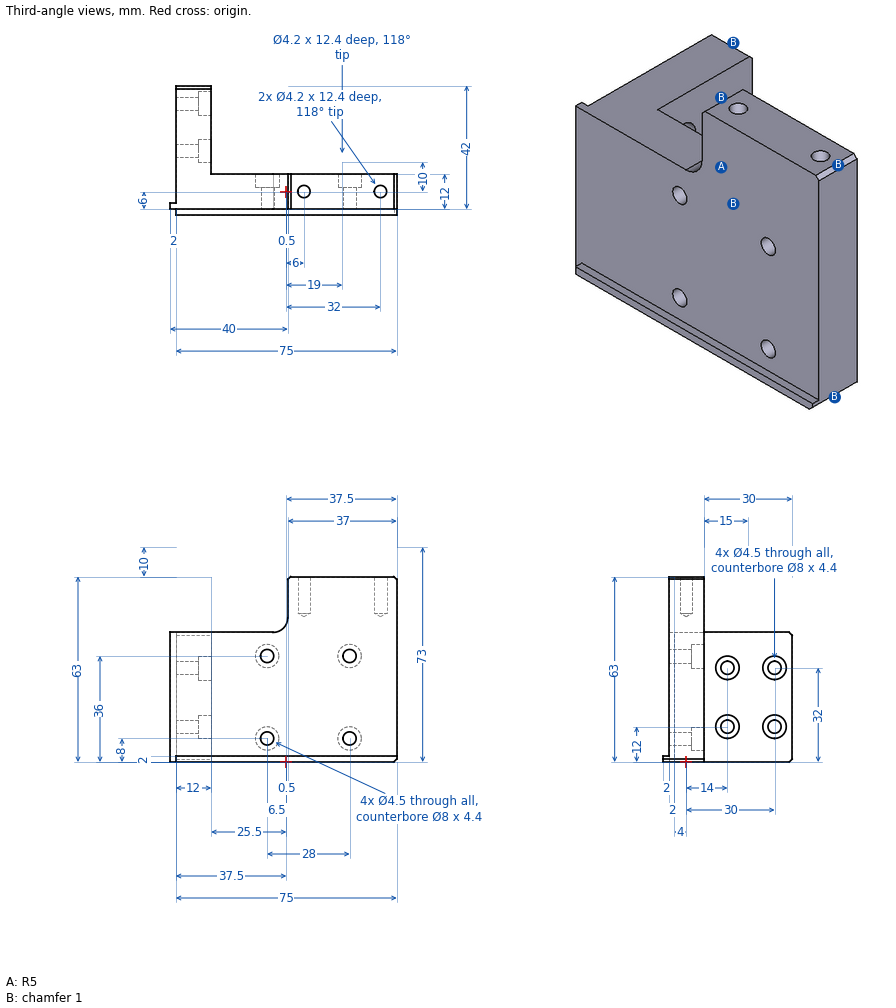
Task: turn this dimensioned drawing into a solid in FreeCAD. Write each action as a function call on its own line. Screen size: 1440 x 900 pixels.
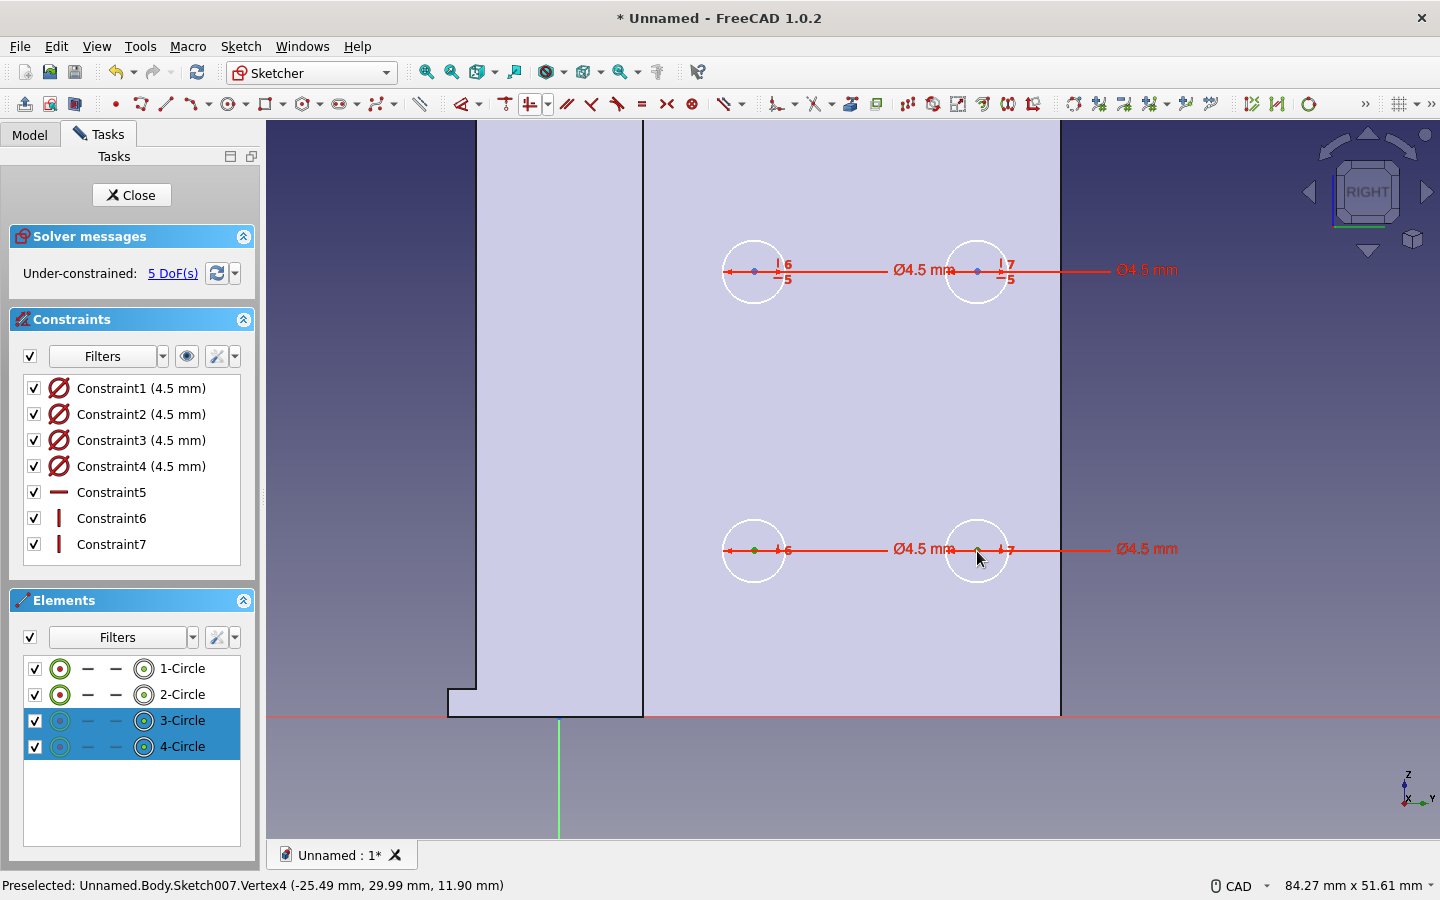
key(h)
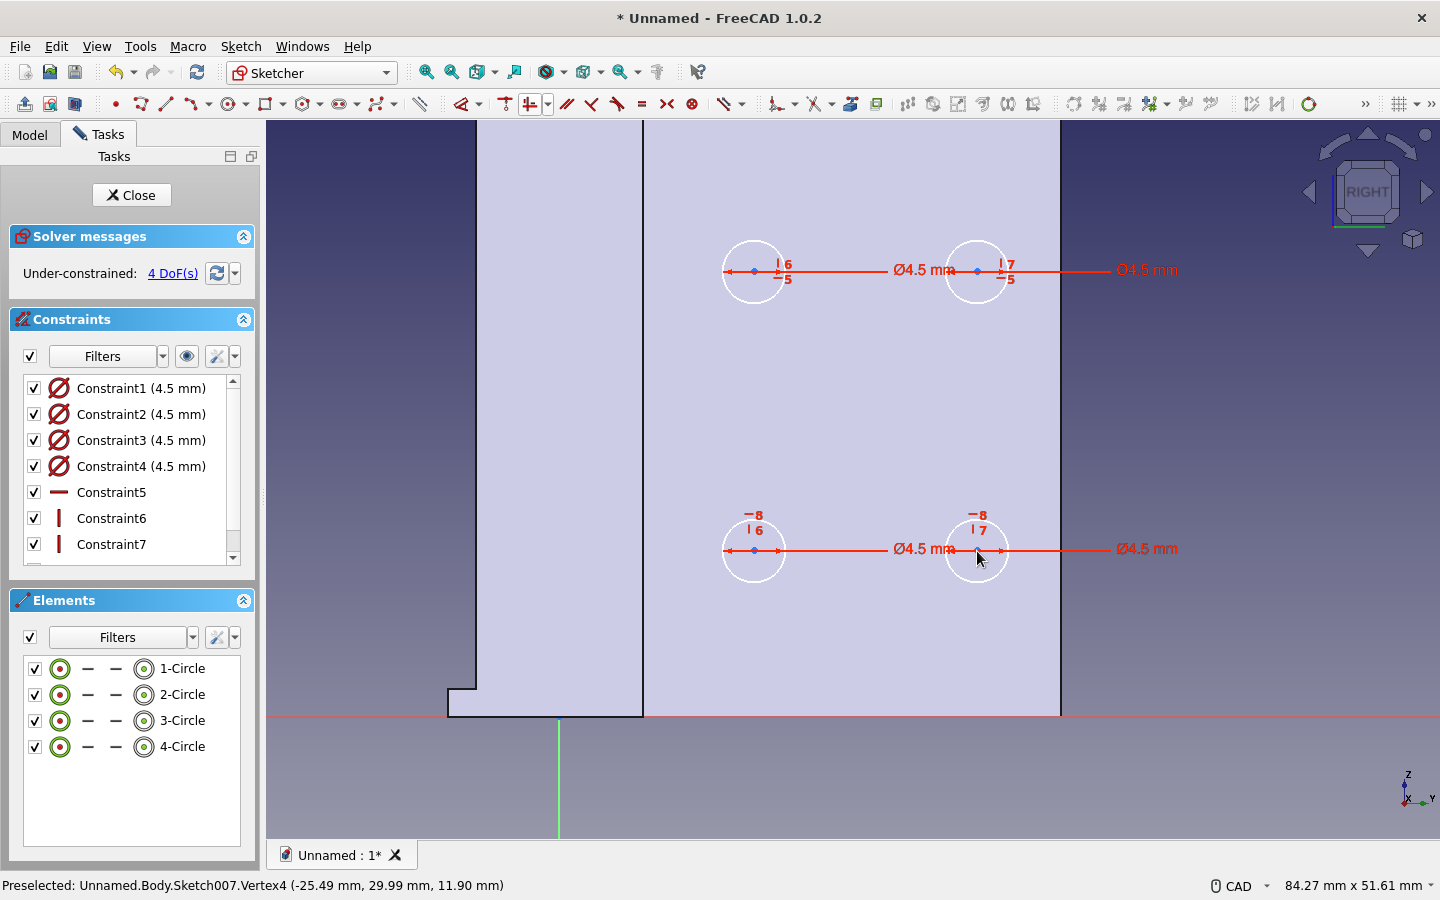
click(460, 104)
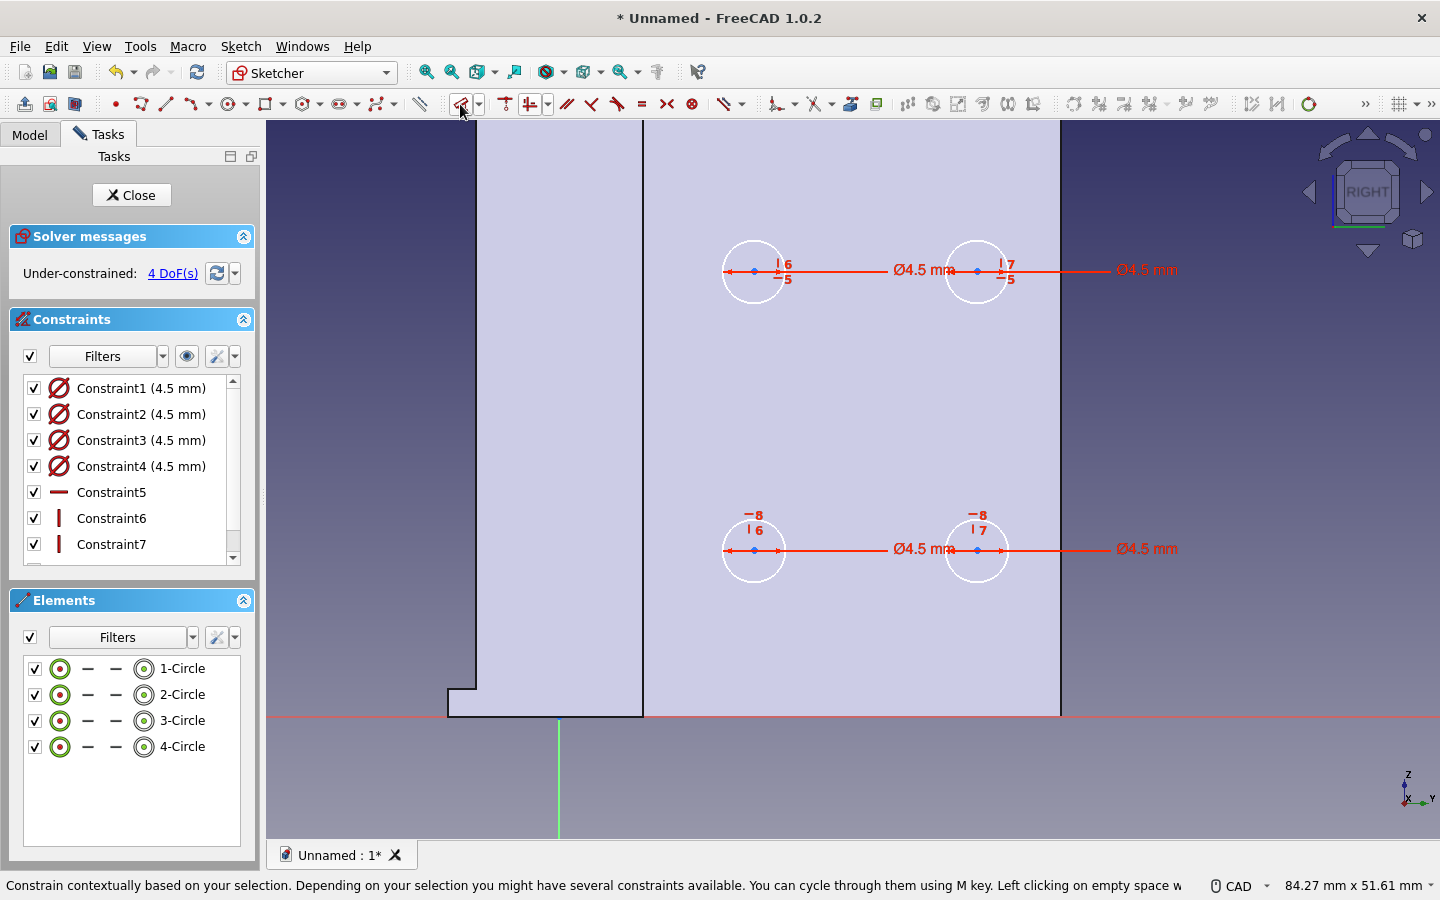
click(977, 272)
click(768, 751)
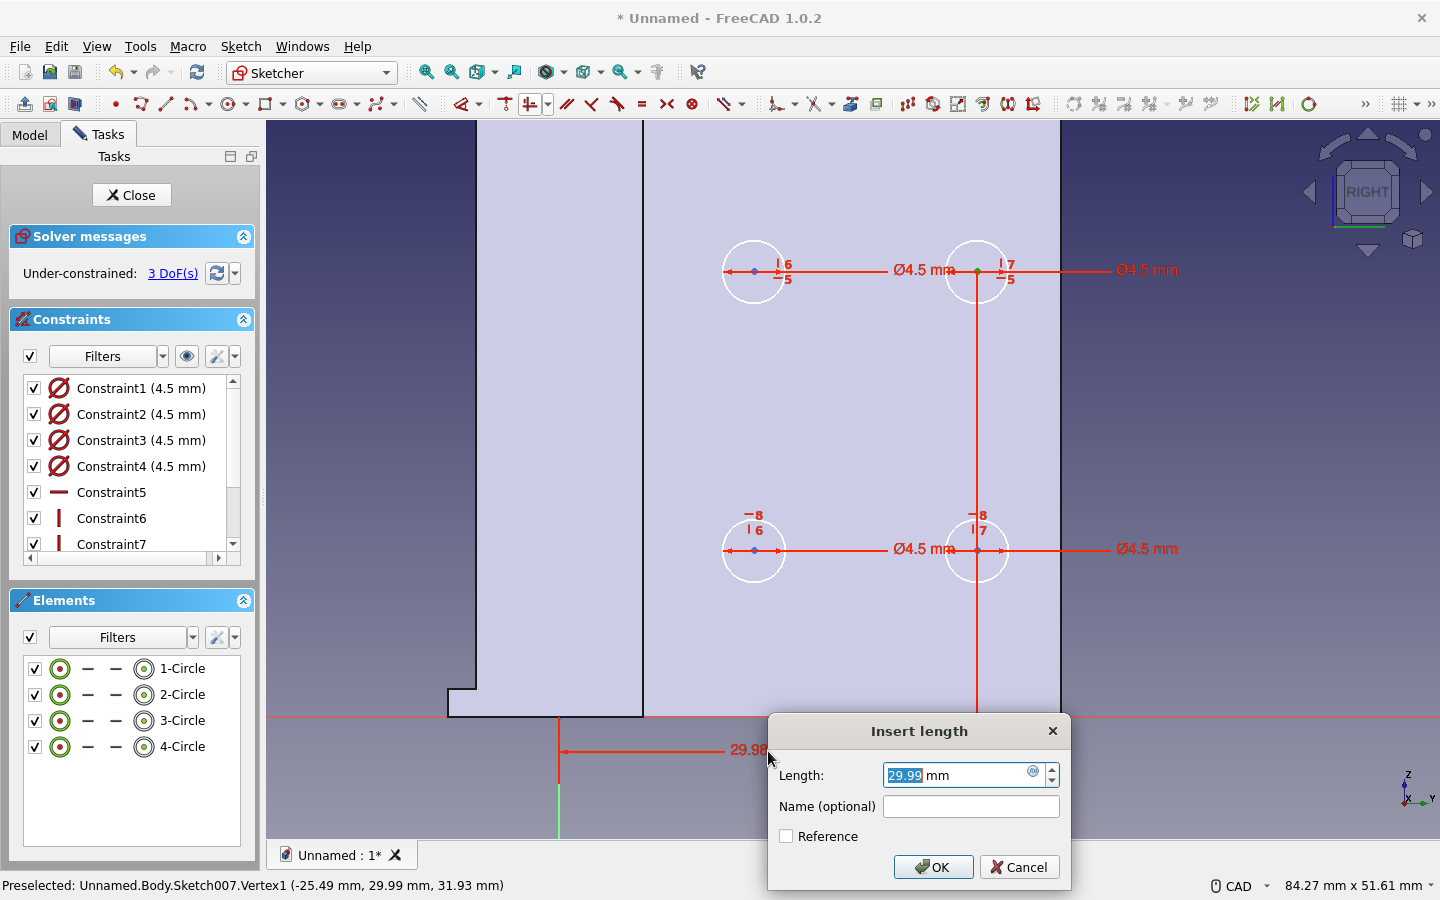
text(30)
key(Return)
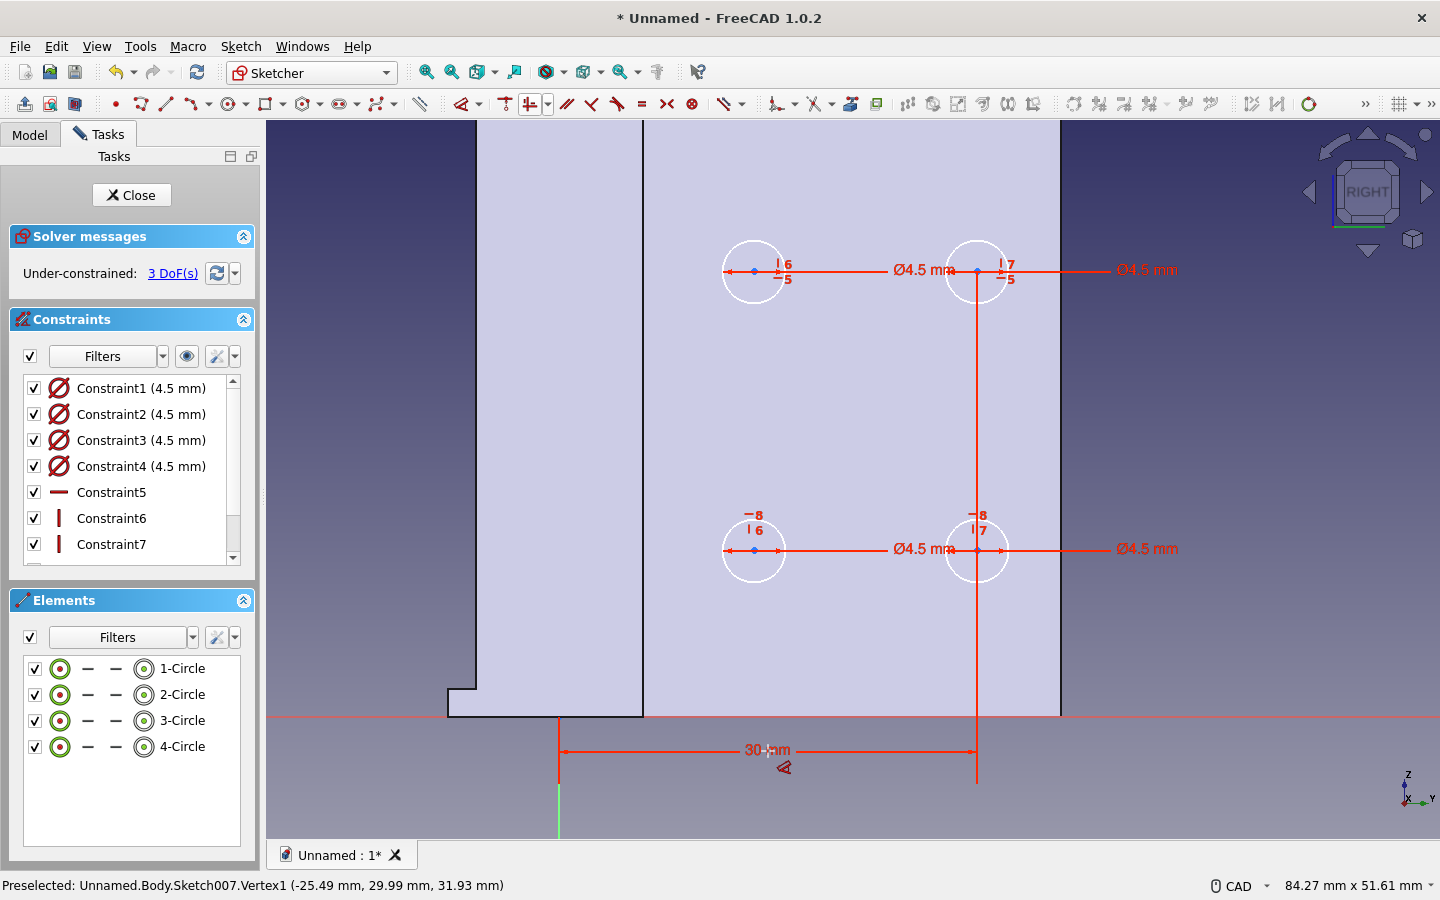
click(977, 272)
click(525, 494)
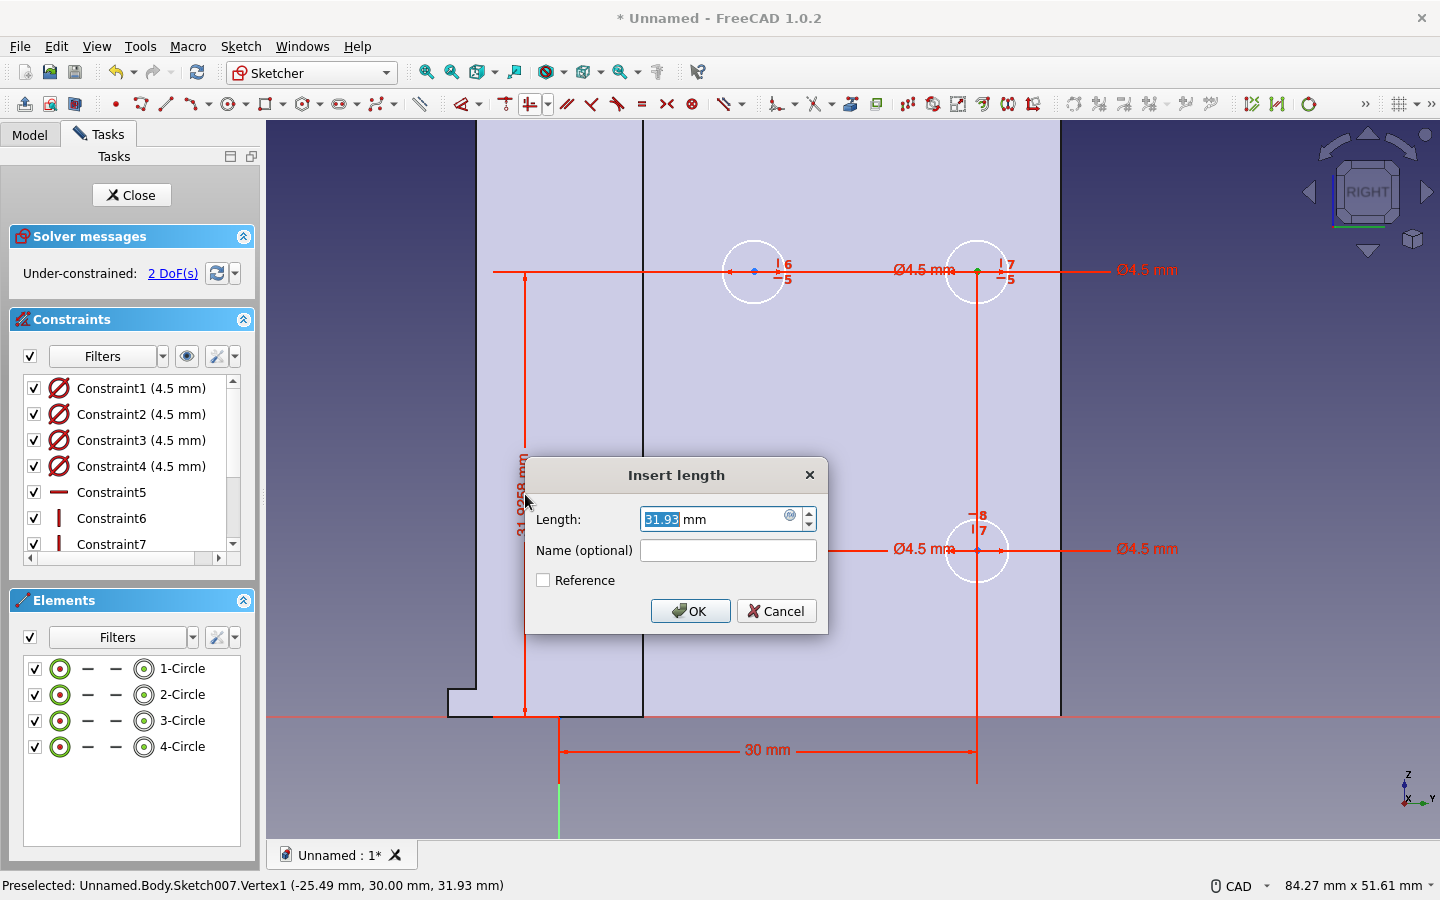
text(32)
key(Return)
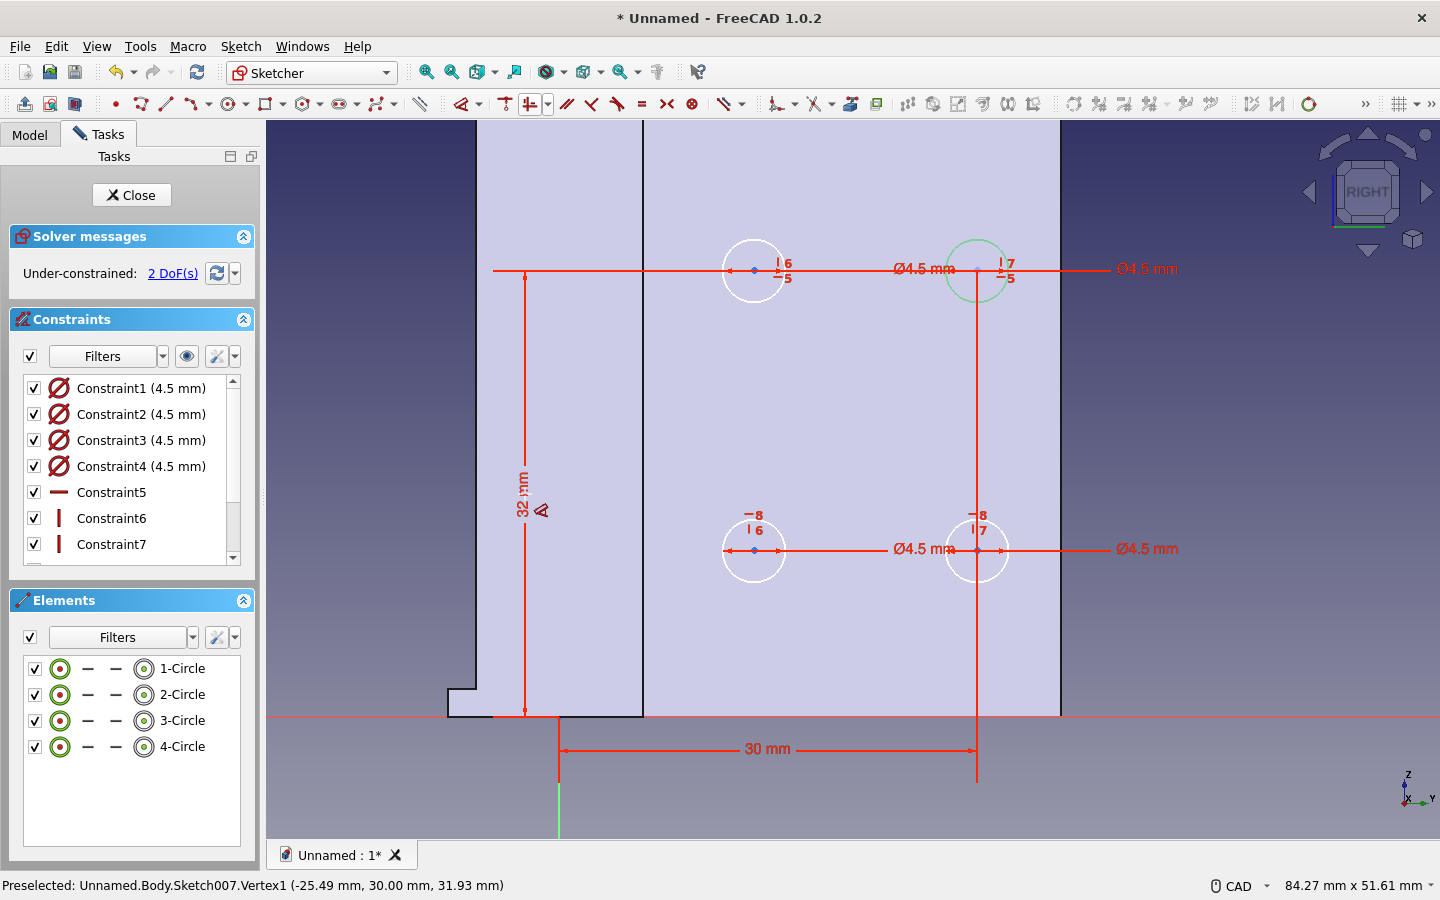
click(754, 271)
click(657, 751)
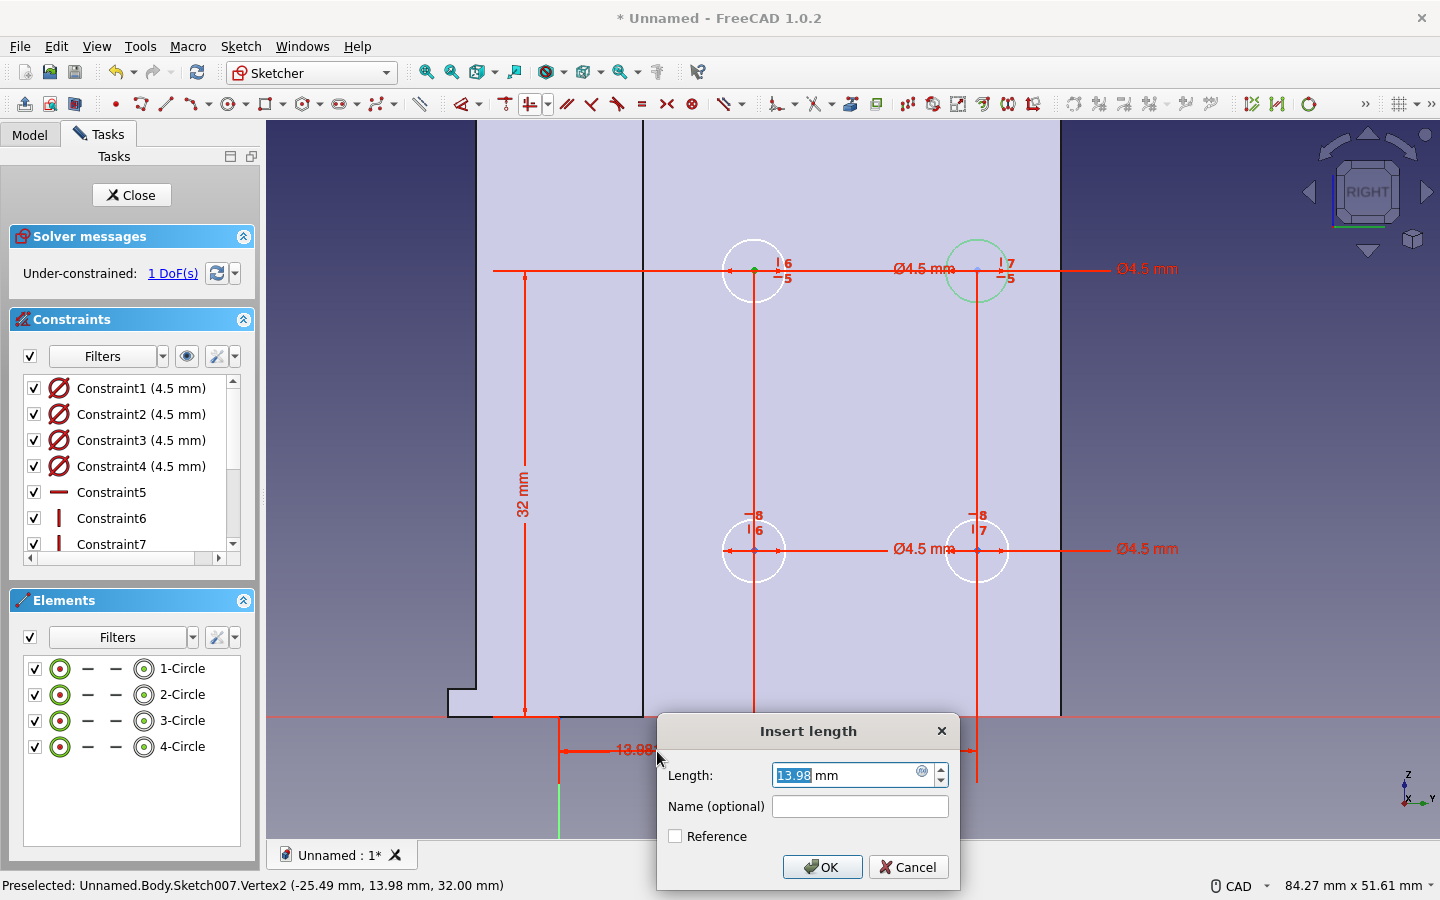
text(14)
key(Return)